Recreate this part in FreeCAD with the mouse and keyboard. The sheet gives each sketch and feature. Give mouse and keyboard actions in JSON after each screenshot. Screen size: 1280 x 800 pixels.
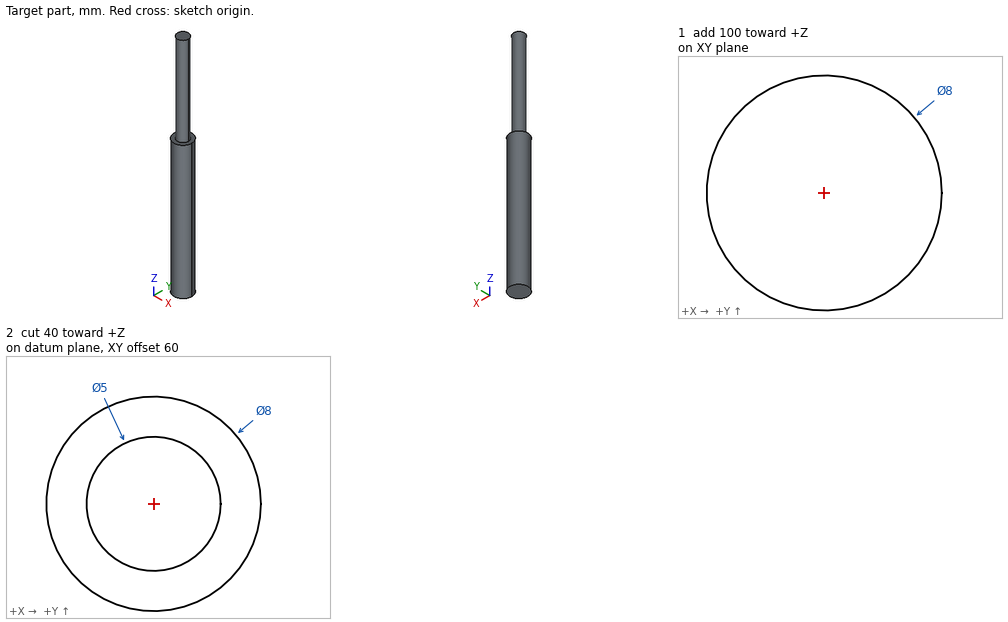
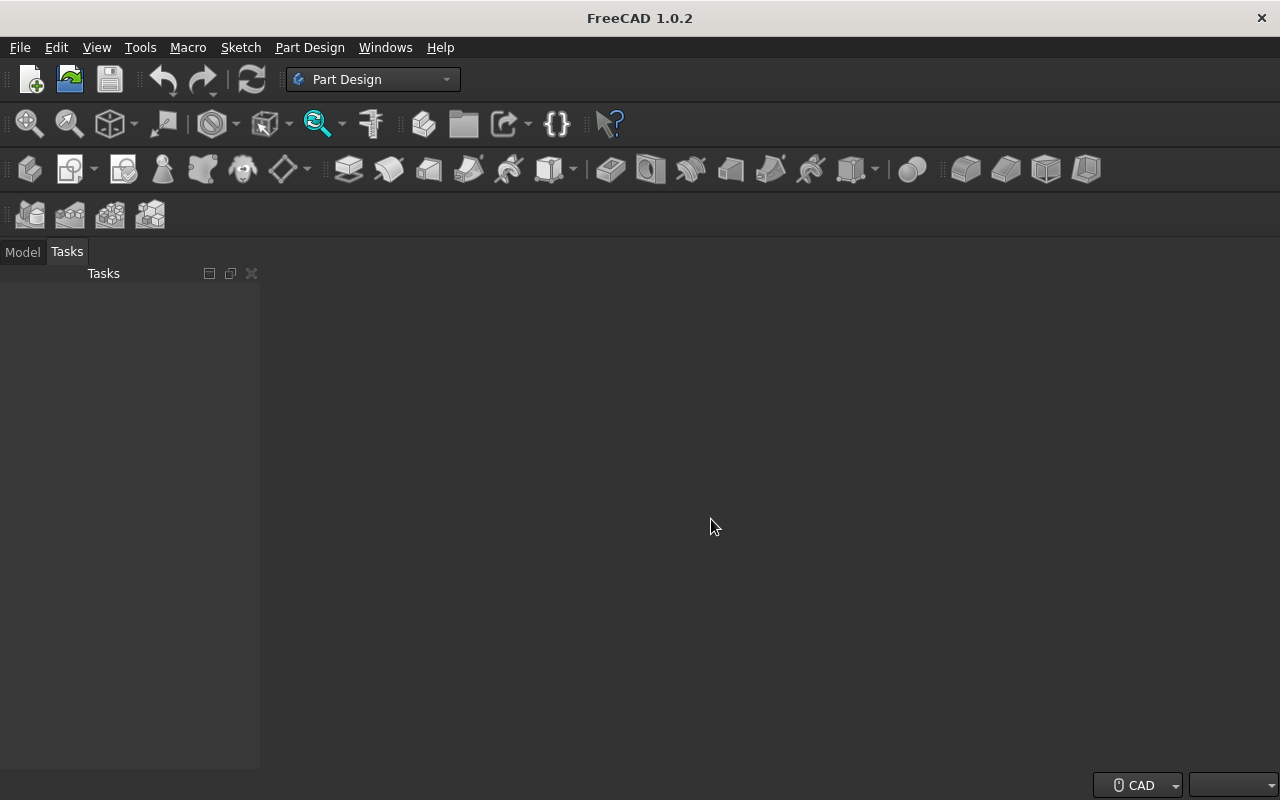
{"action": "left_click", "coordinate": [30, 80]}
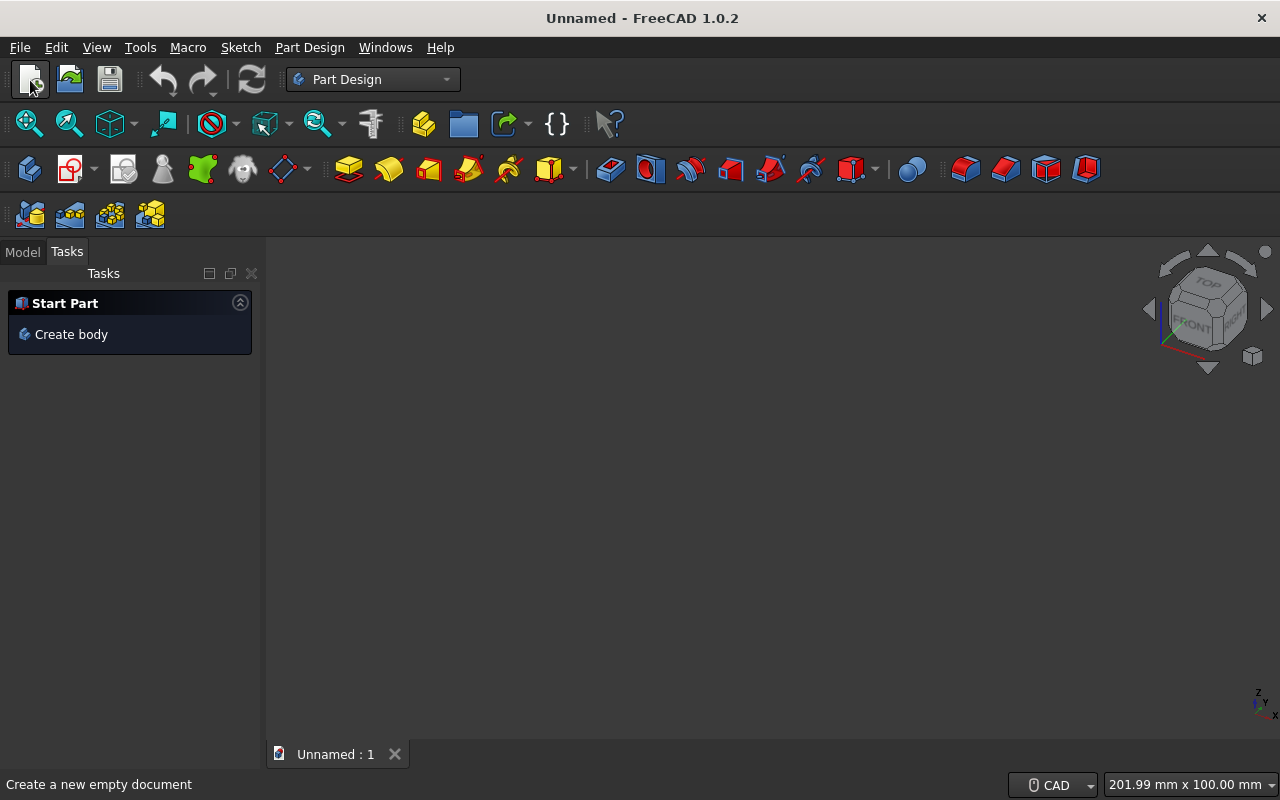
{"action": "left_click", "coordinate": [70, 170]}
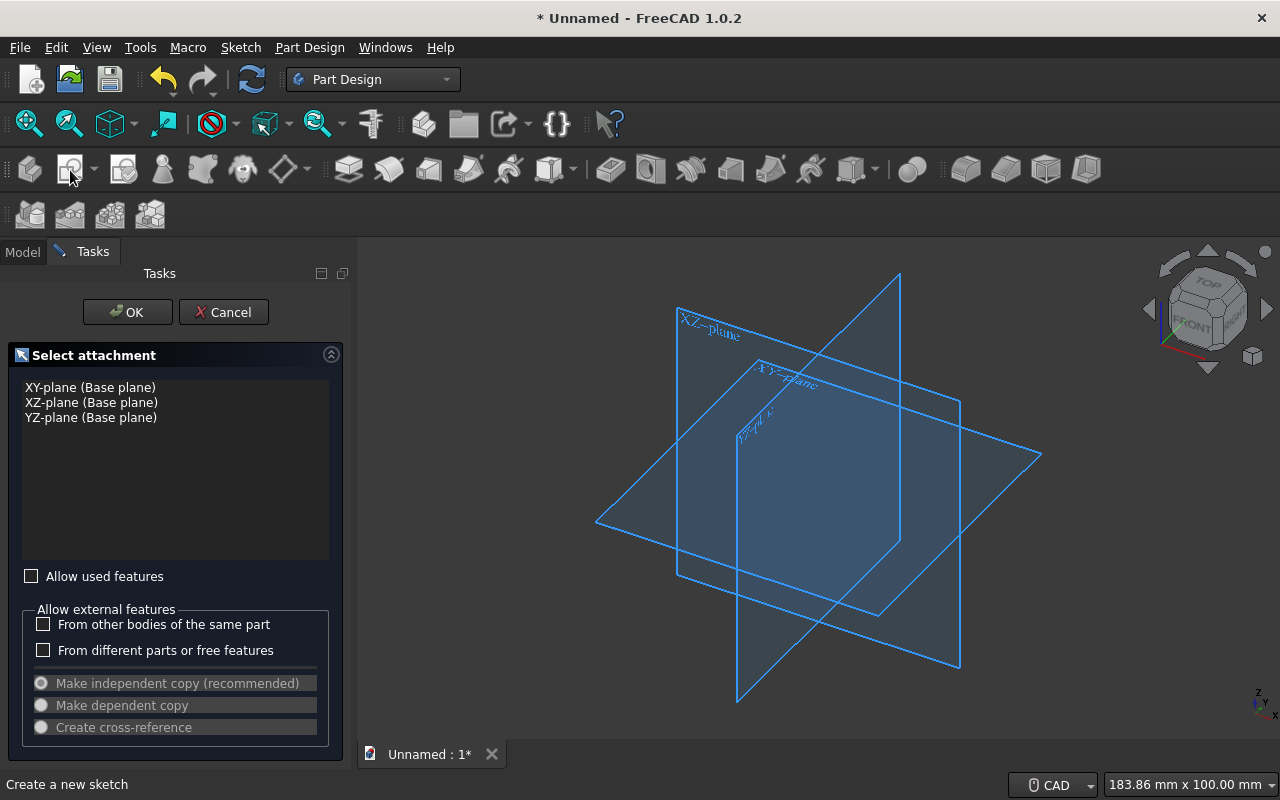
{"action": "left_click", "coordinate": [82, 388]}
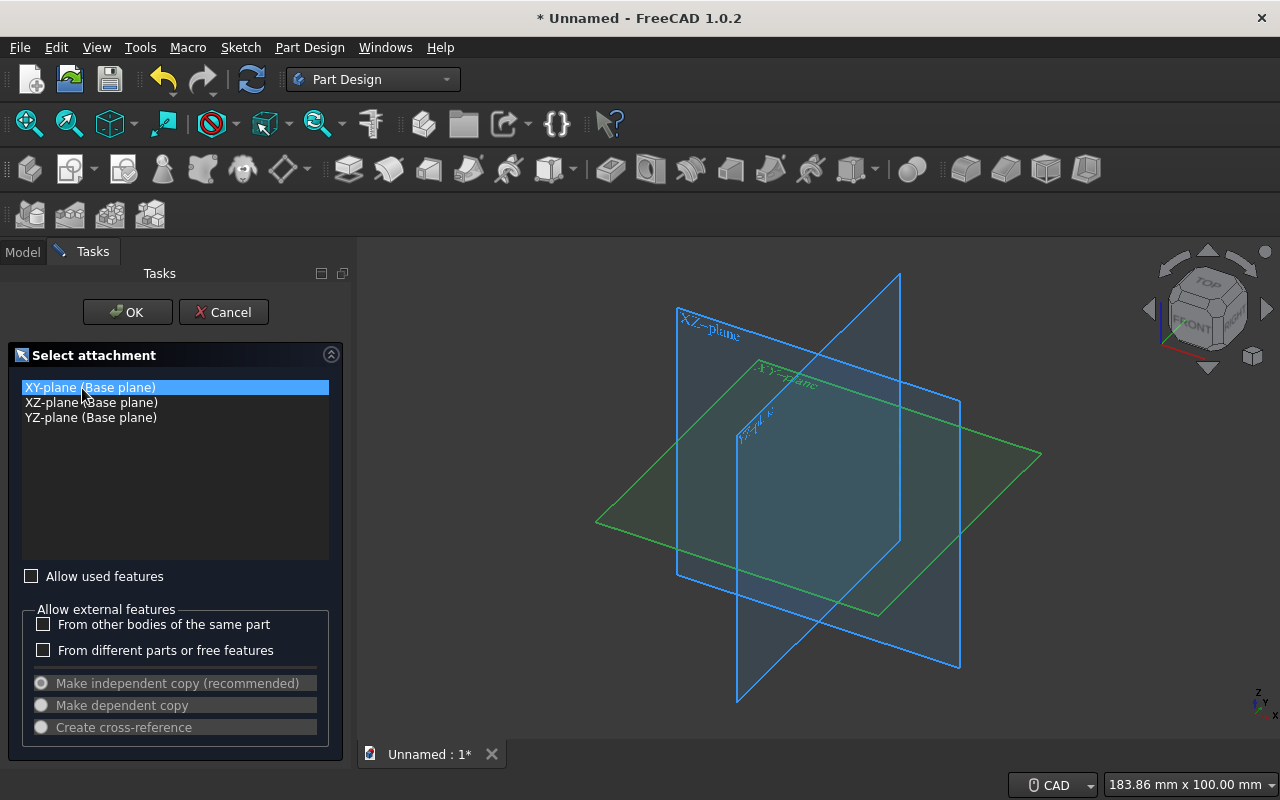
{"action": "left_click", "coordinate": [128, 312]}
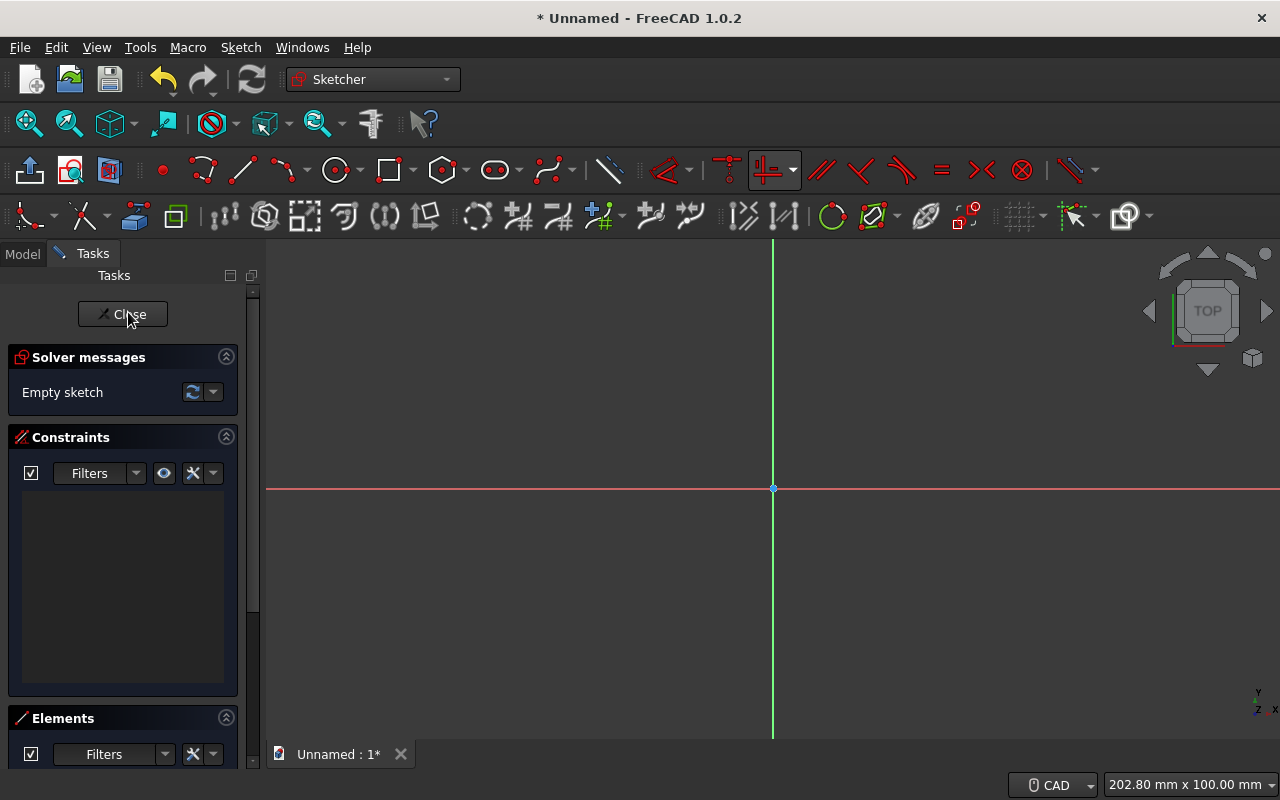
{"action": "scroll", "coordinate": [784, 489], "scroll_direction": "up", "scroll_amount": 10}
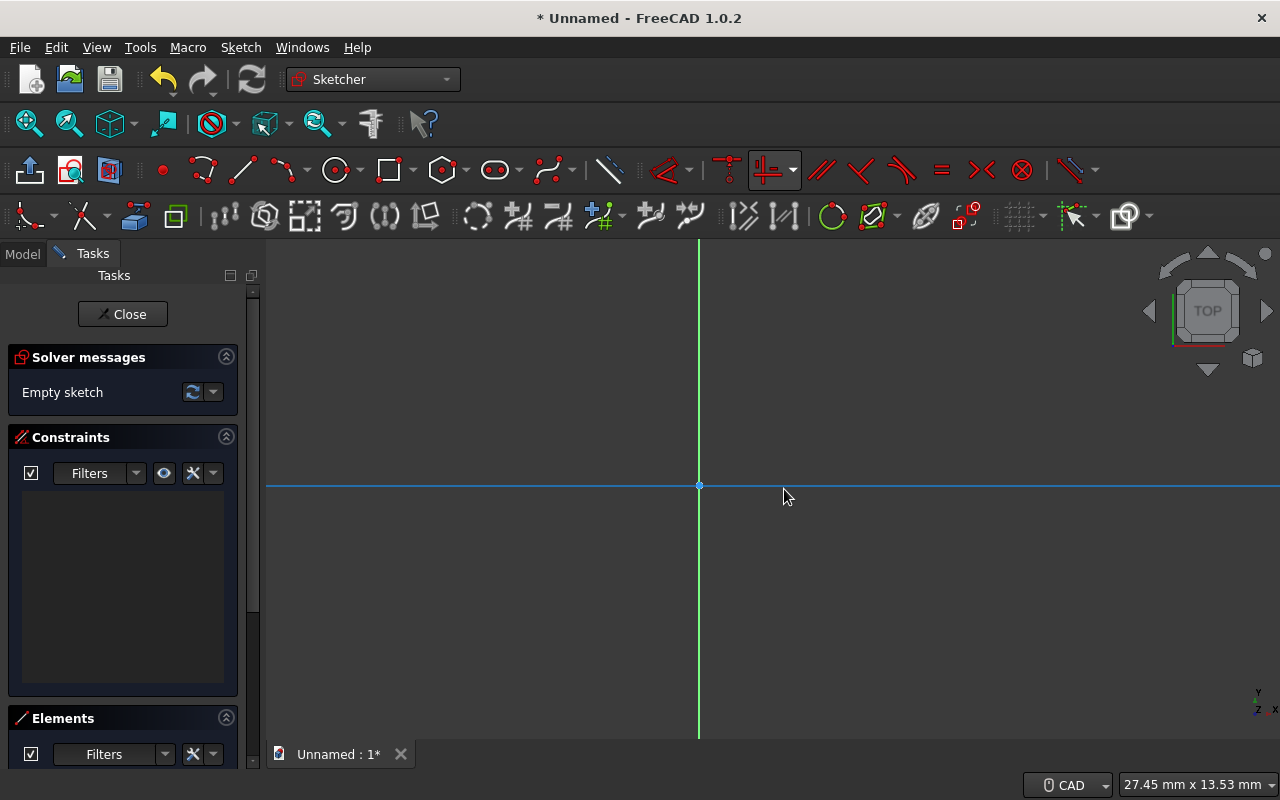
{"action": "left_click", "coordinate": [336, 170]}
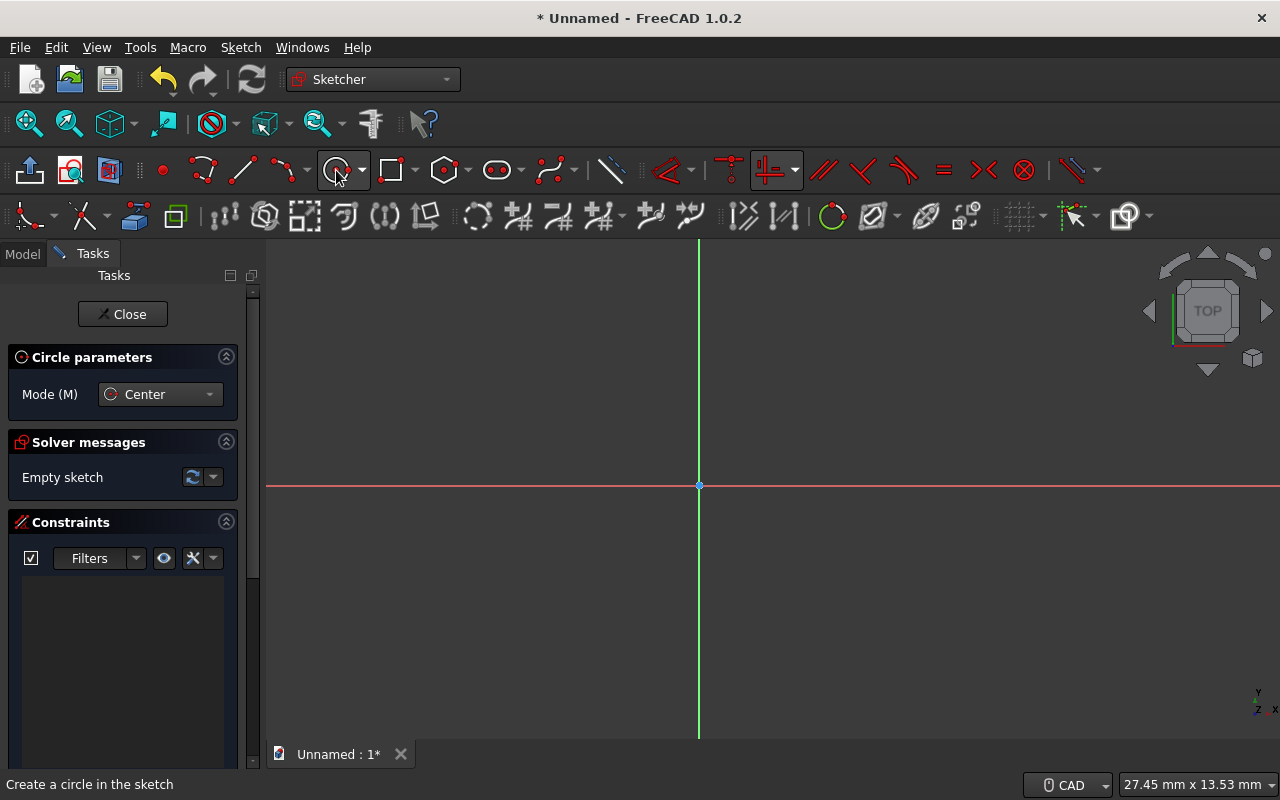
{"action": "left_click", "coordinate": [699, 486]}
{"action": "mouse_move", "coordinate": [804, 381]}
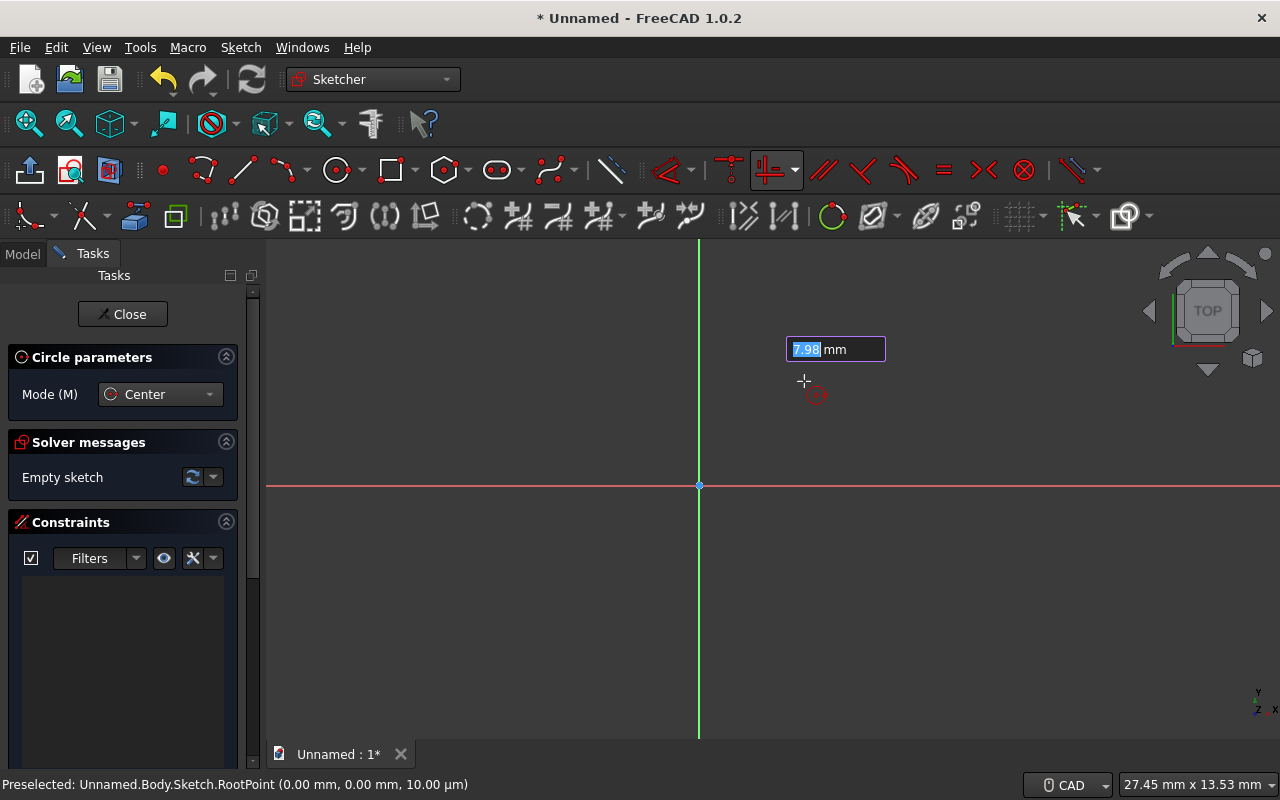
{"action": "type", "text": "8"}
{"action": "key", "text": "Return"}
{"action": "key", "text": "Escape"}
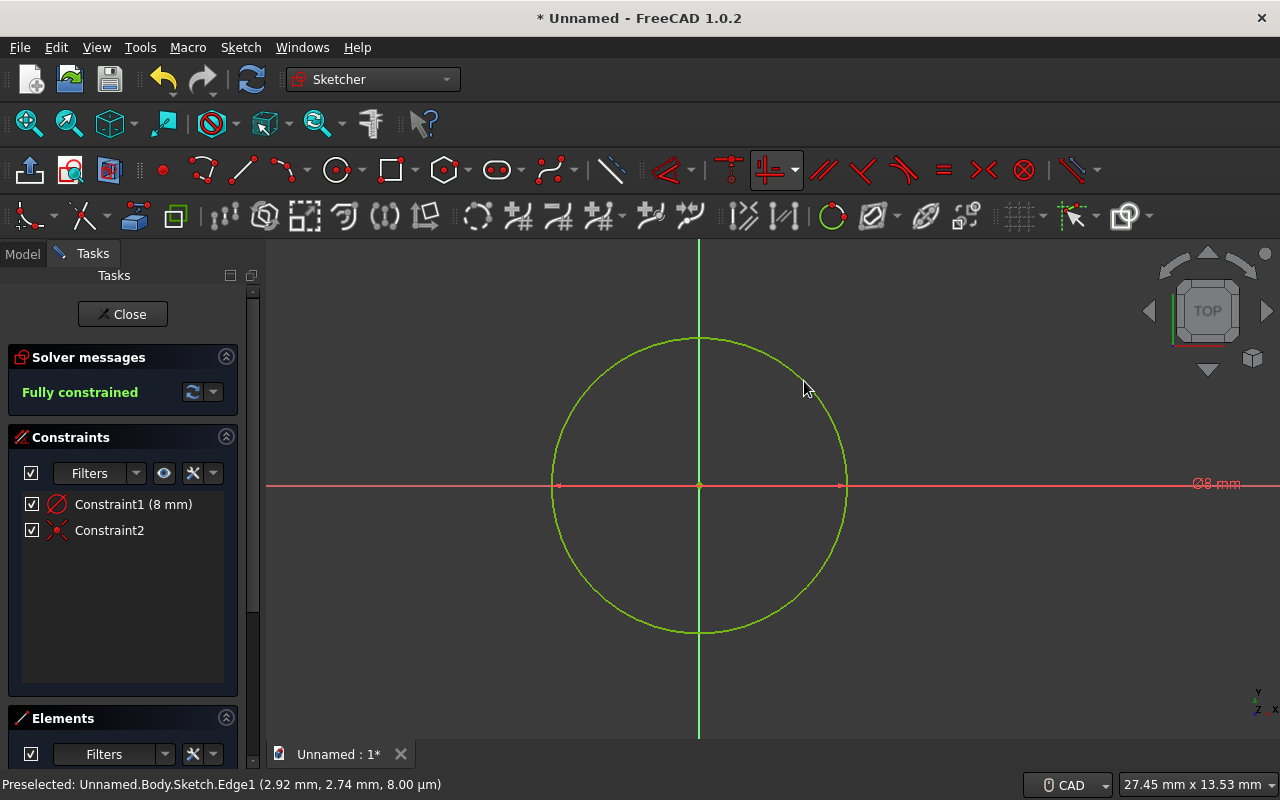
{"action": "left_click", "coordinate": [123, 314]}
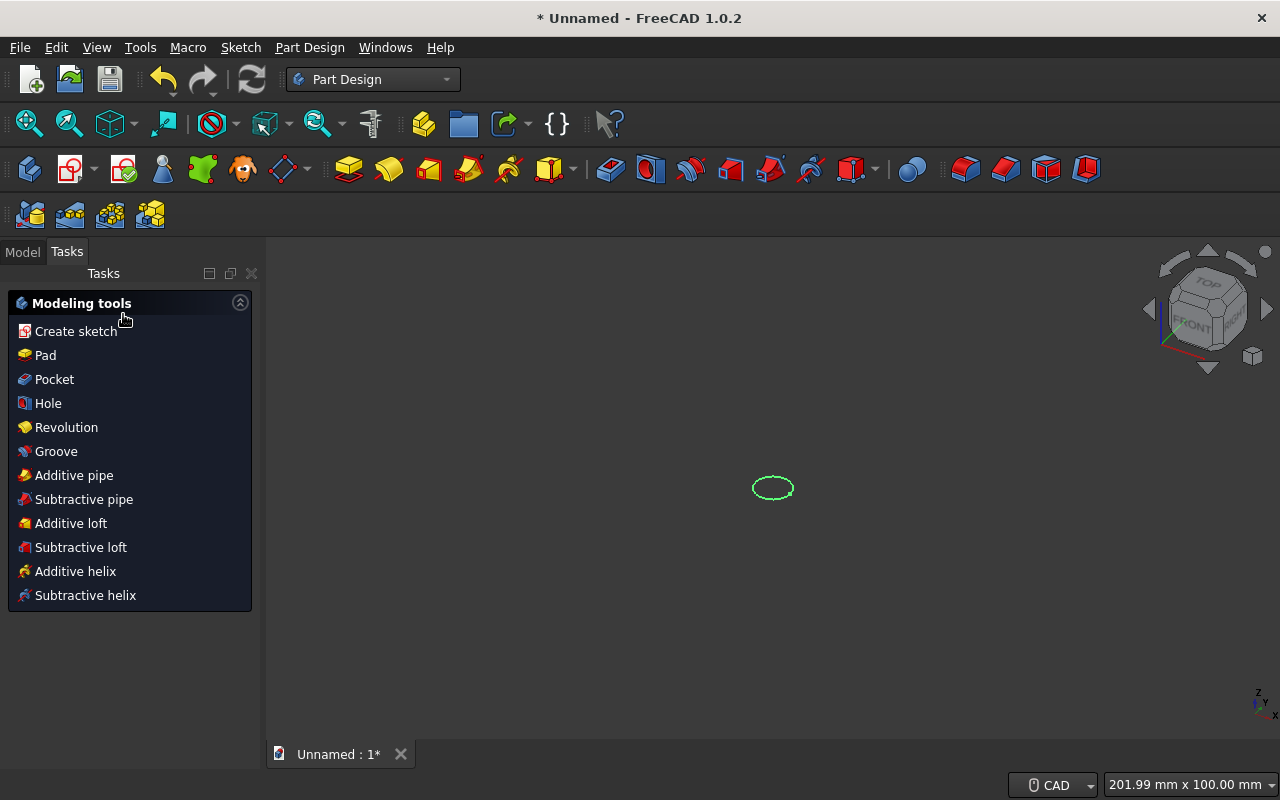
{"action": "left_click", "coordinate": [350, 170]}